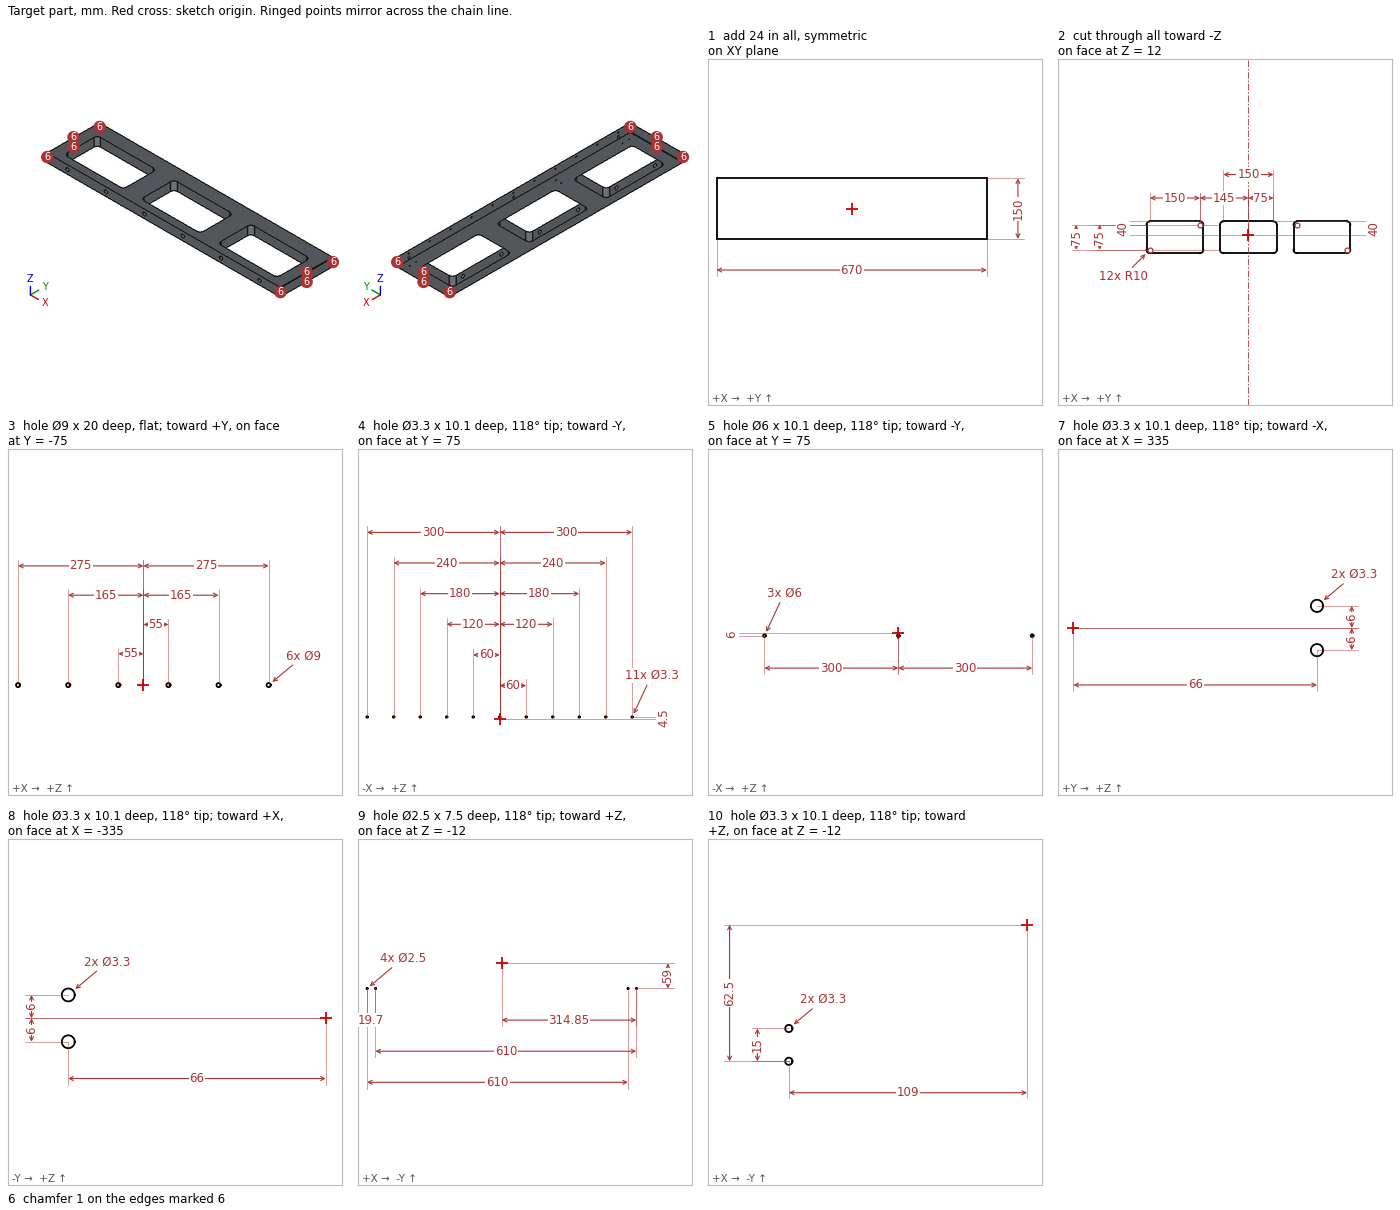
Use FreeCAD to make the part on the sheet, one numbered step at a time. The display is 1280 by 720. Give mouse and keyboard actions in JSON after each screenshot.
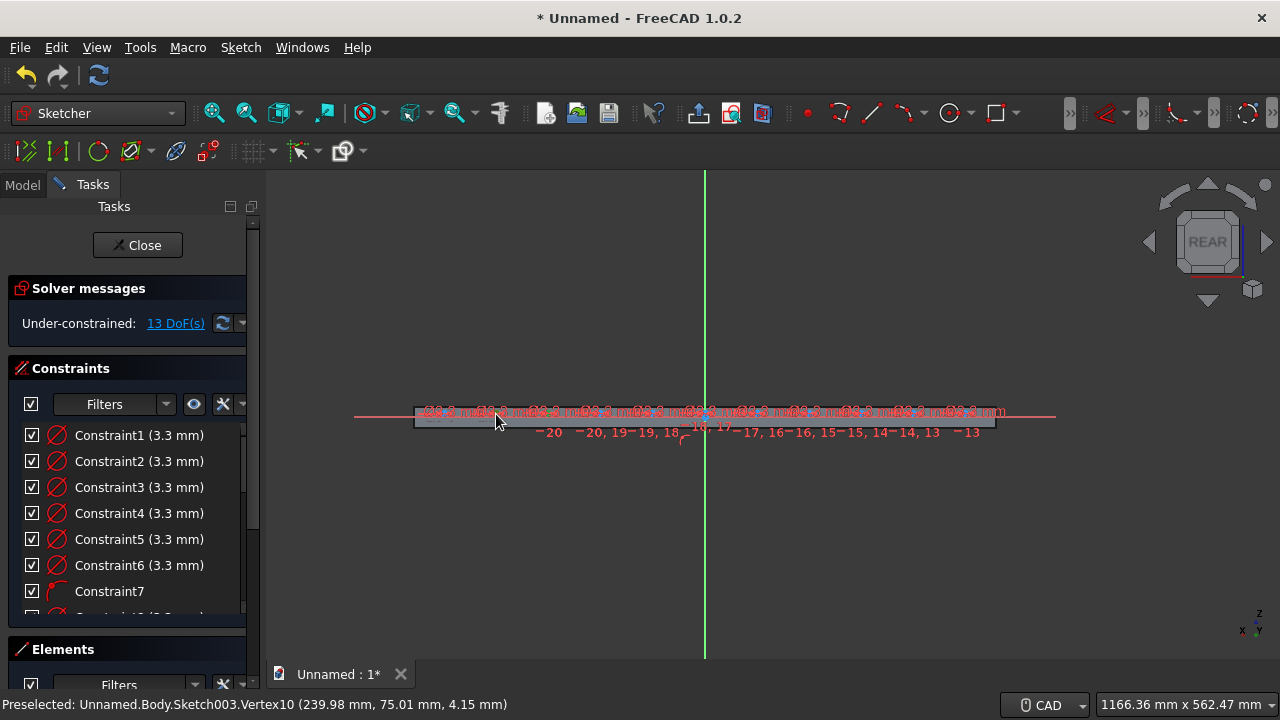
{"action": "key", "text": "h"}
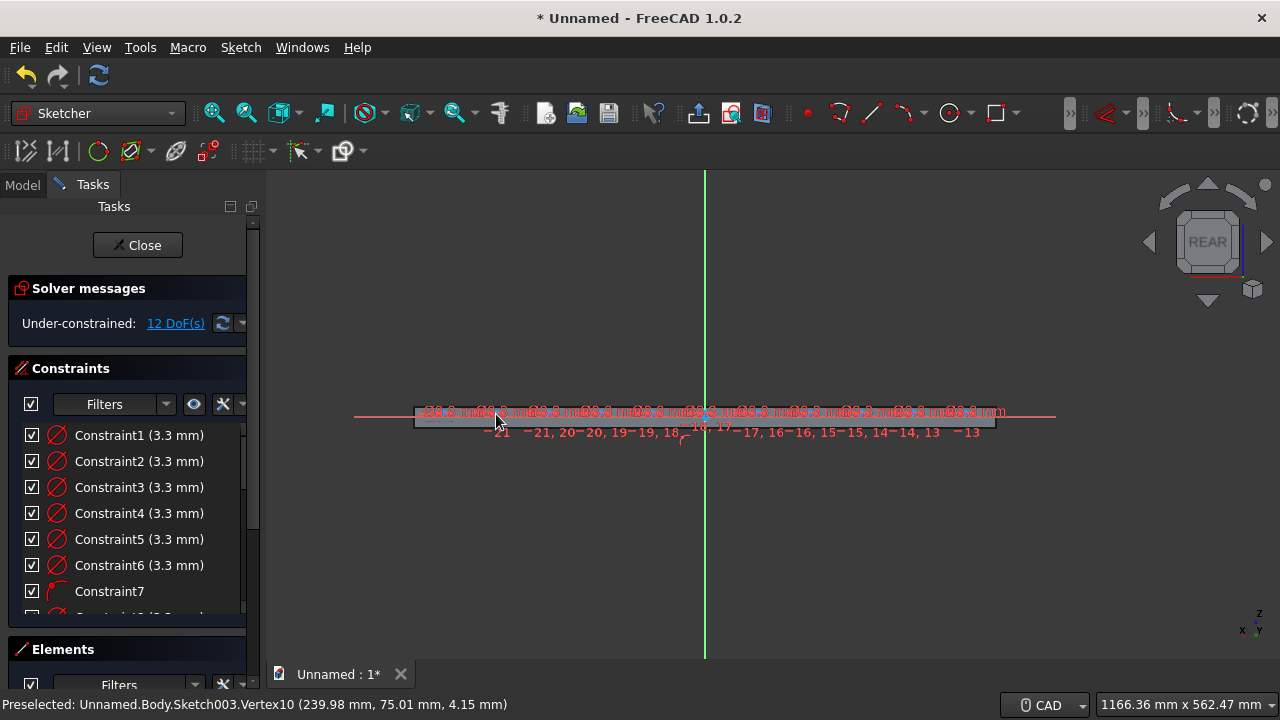
{"action": "left_click", "coordinate": [496, 413]}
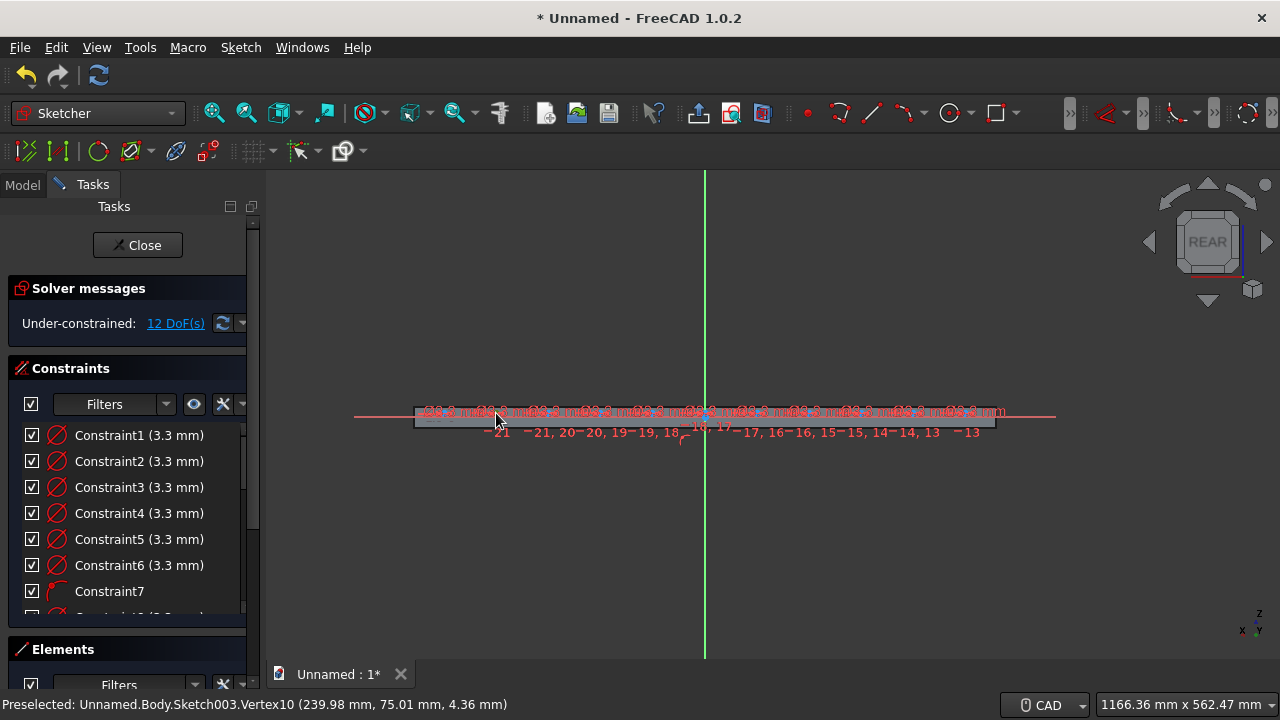
{"action": "left_click", "coordinate": [444, 414]}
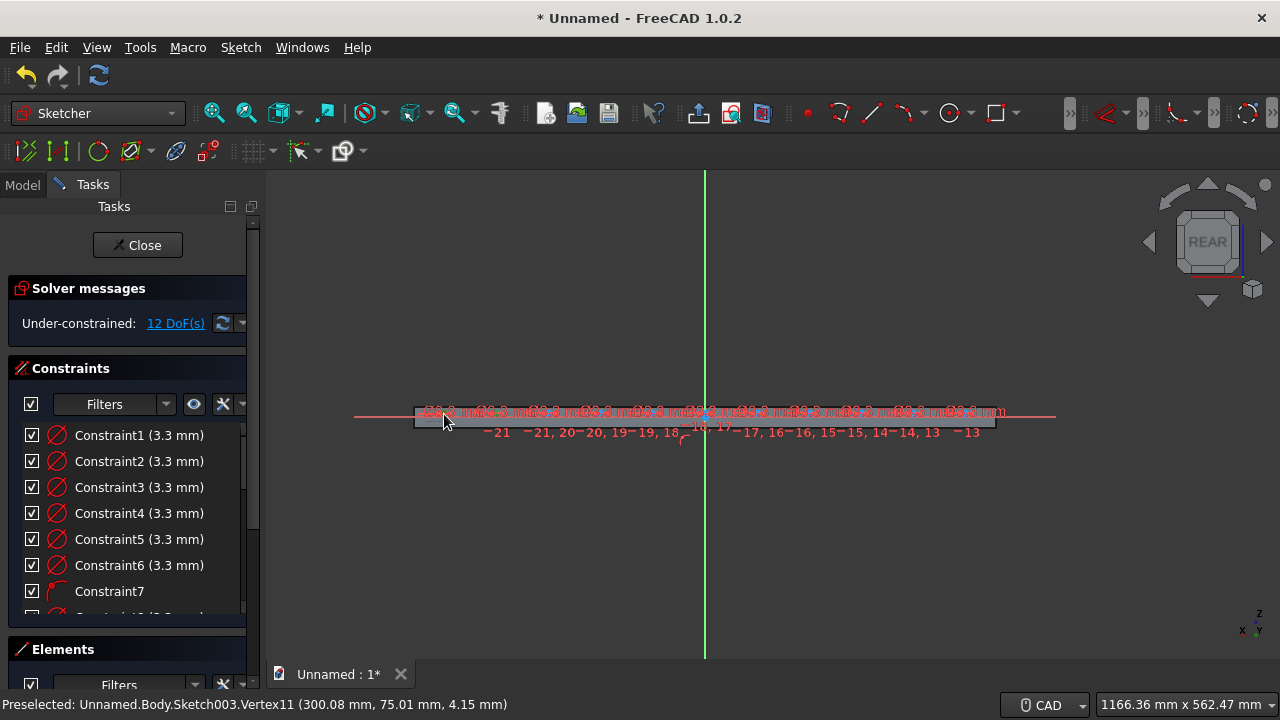
{"action": "key", "text": "h"}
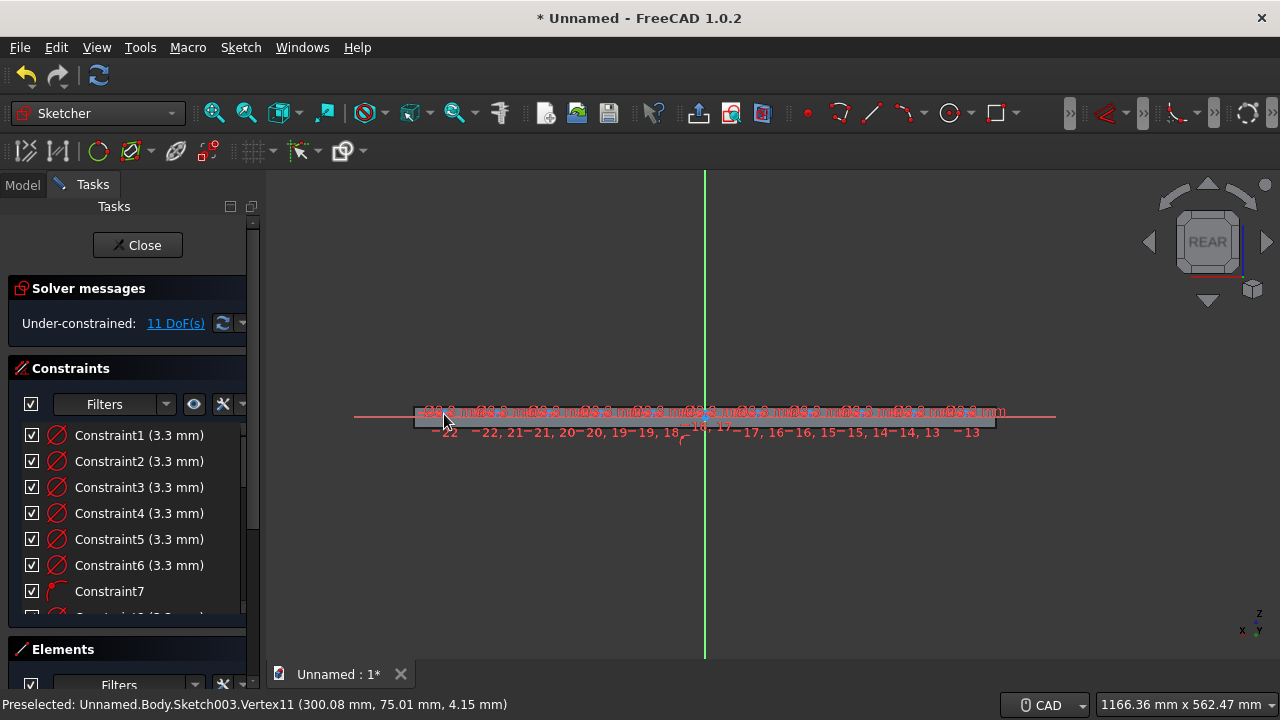
{"action": "left_click", "coordinate": [1106, 114]}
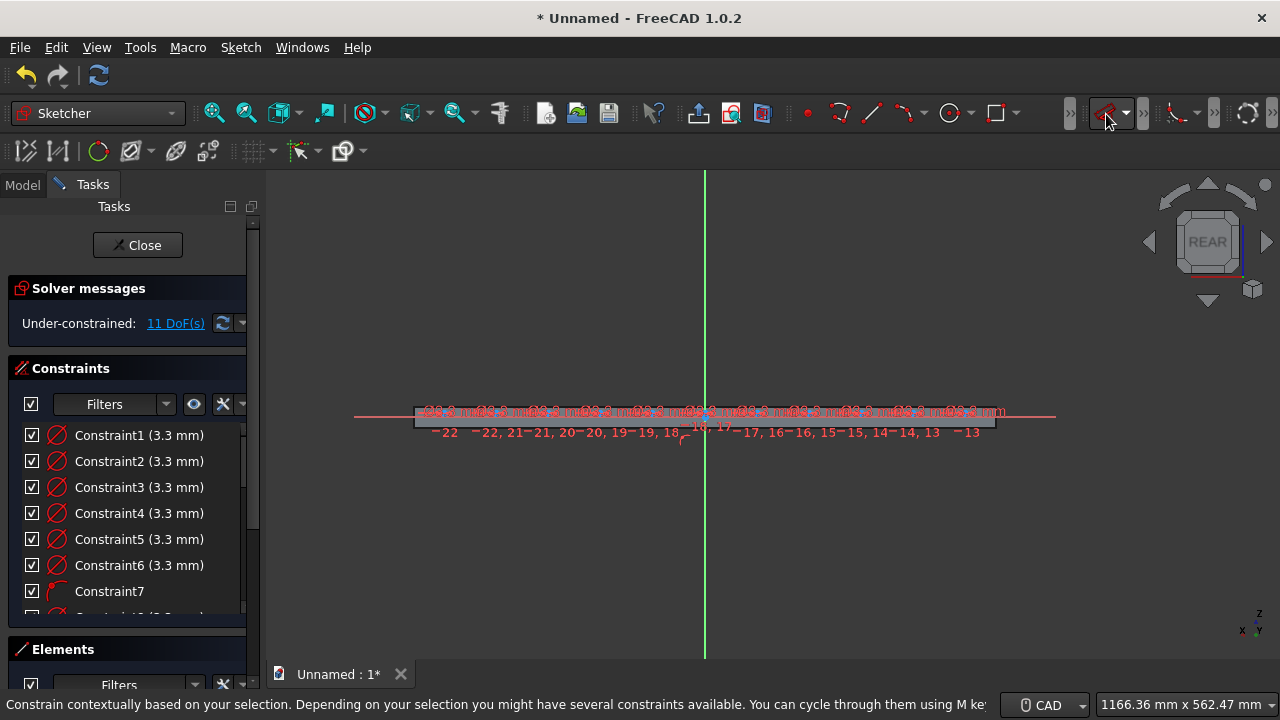
{"action": "left_click", "coordinate": [757, 413]}
{"action": "left_click", "coordinate": [731, 451]}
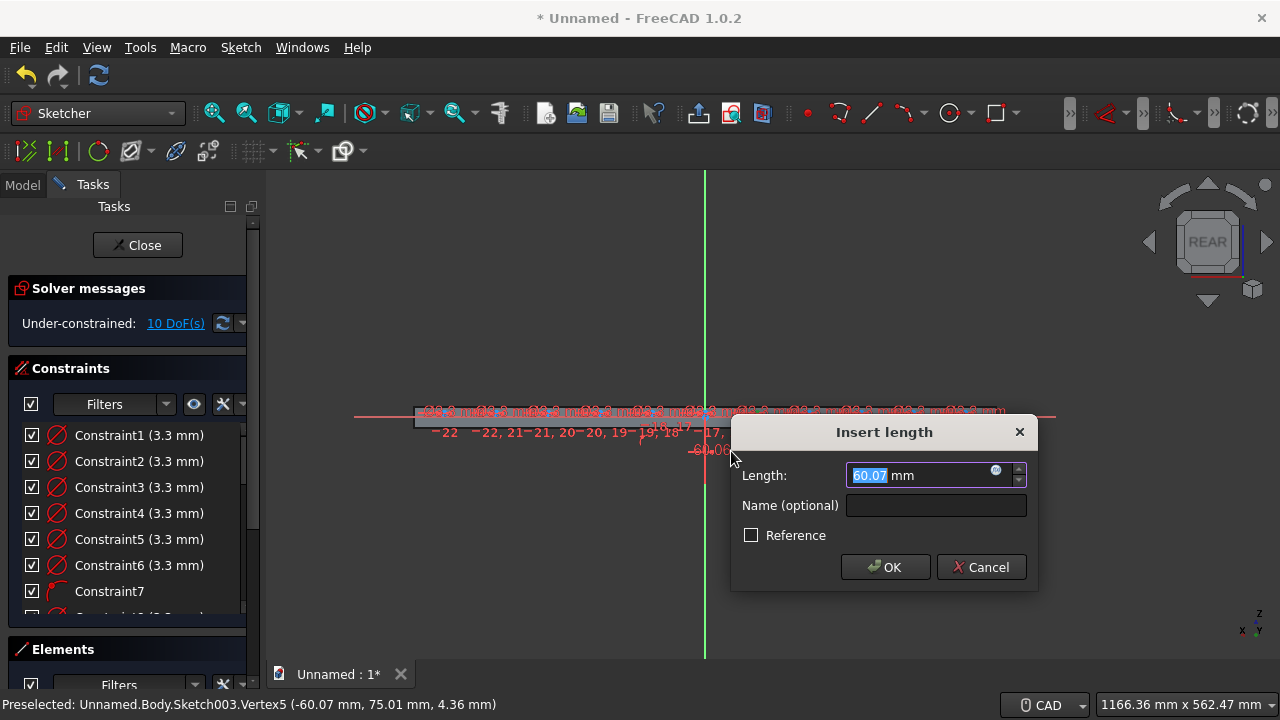
{"action": "type", "text": "60"}
{"action": "key", "text": "Return"}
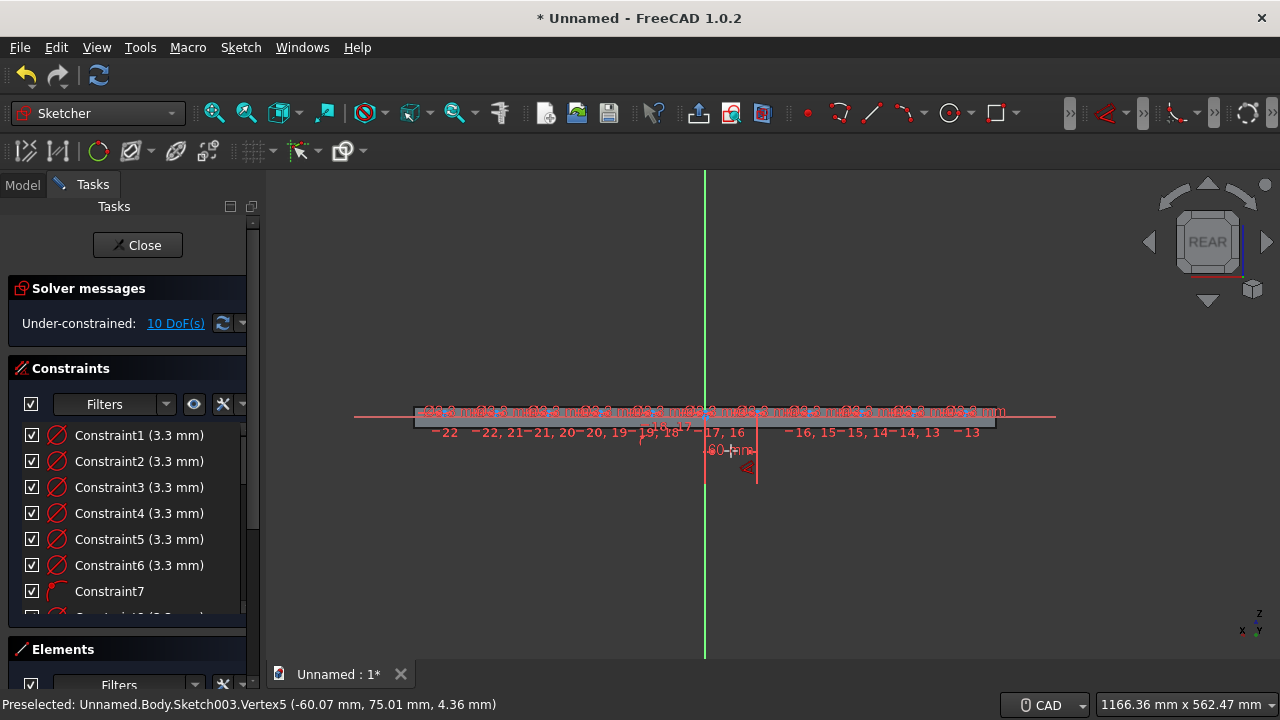
{"action": "left_click", "coordinate": [653, 413]}
{"action": "left_click", "coordinate": [661, 451]}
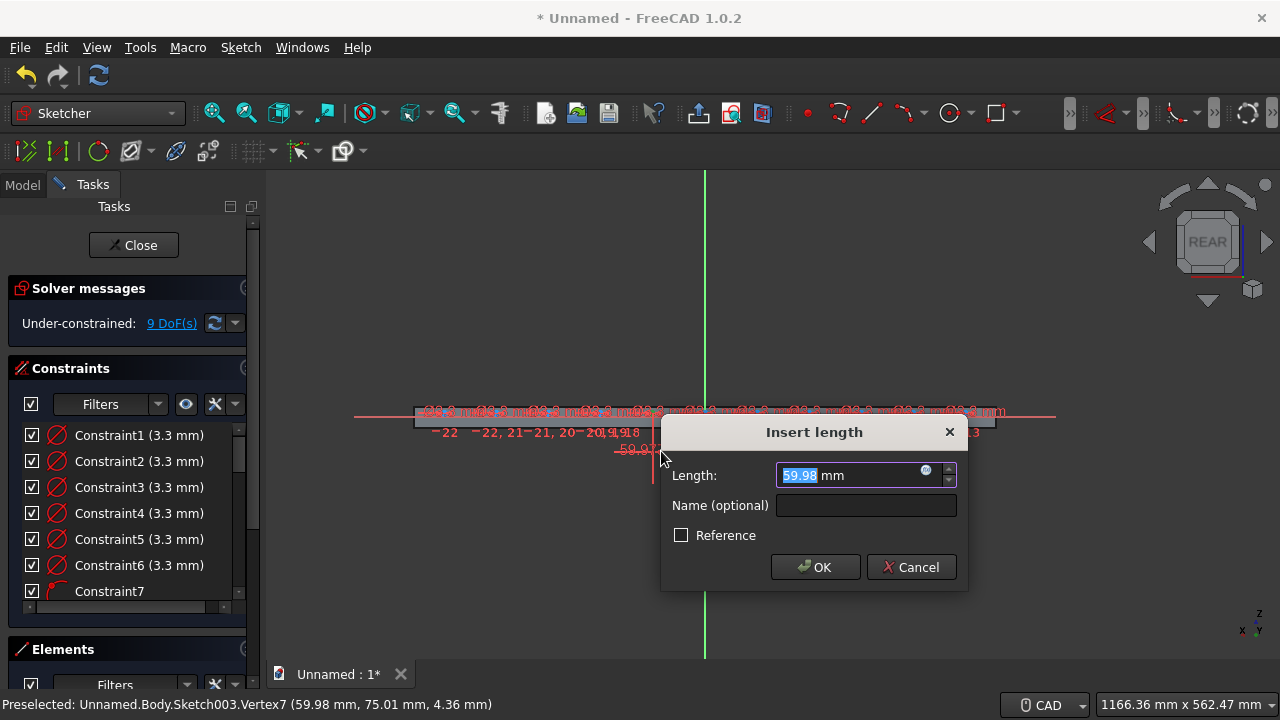
{"action": "type", "text": "60"}
{"action": "key", "text": "Return"}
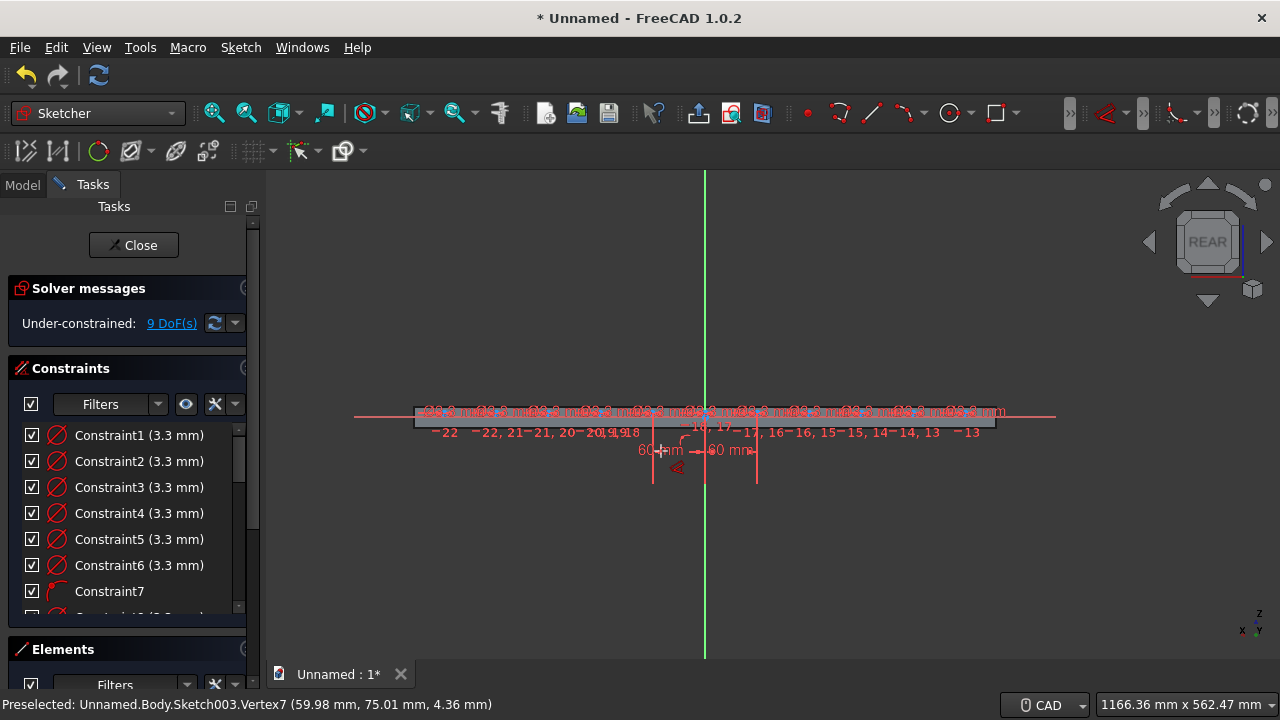
{"action": "left_click", "coordinate": [966, 413]}
{"action": "left_click", "coordinate": [835, 451]}